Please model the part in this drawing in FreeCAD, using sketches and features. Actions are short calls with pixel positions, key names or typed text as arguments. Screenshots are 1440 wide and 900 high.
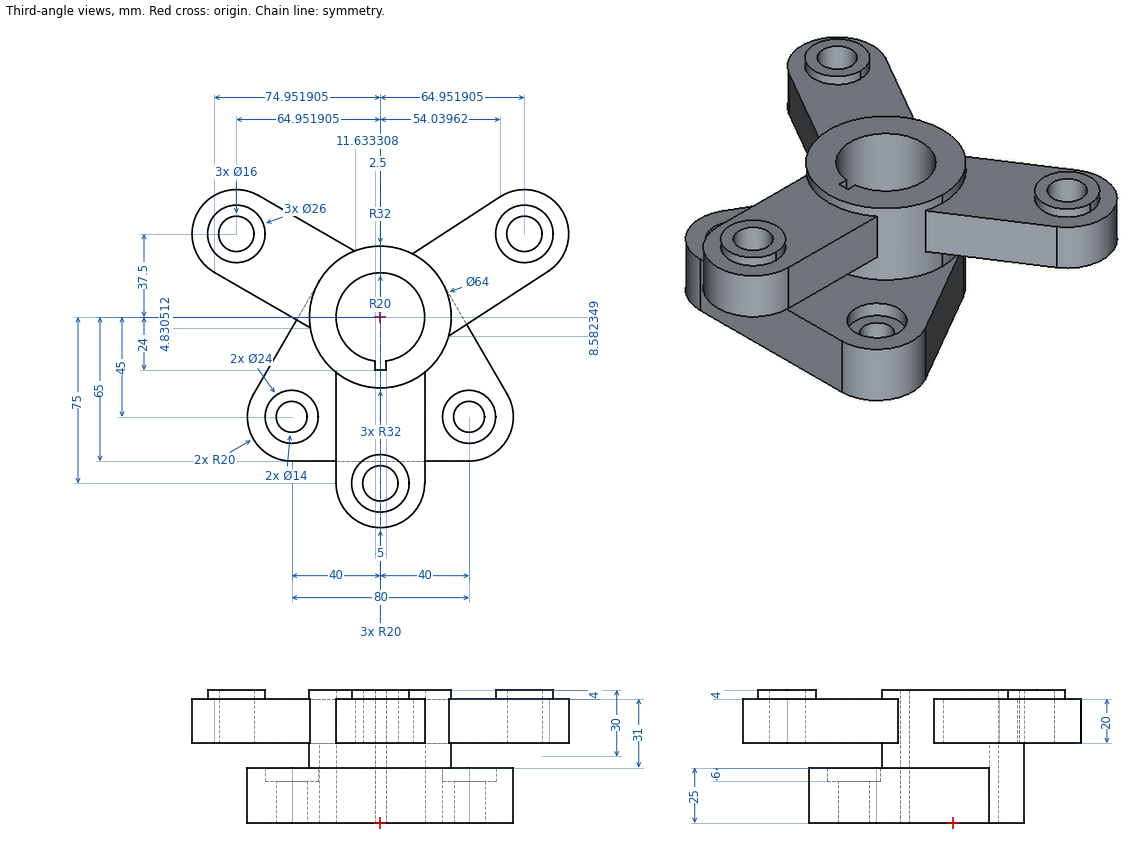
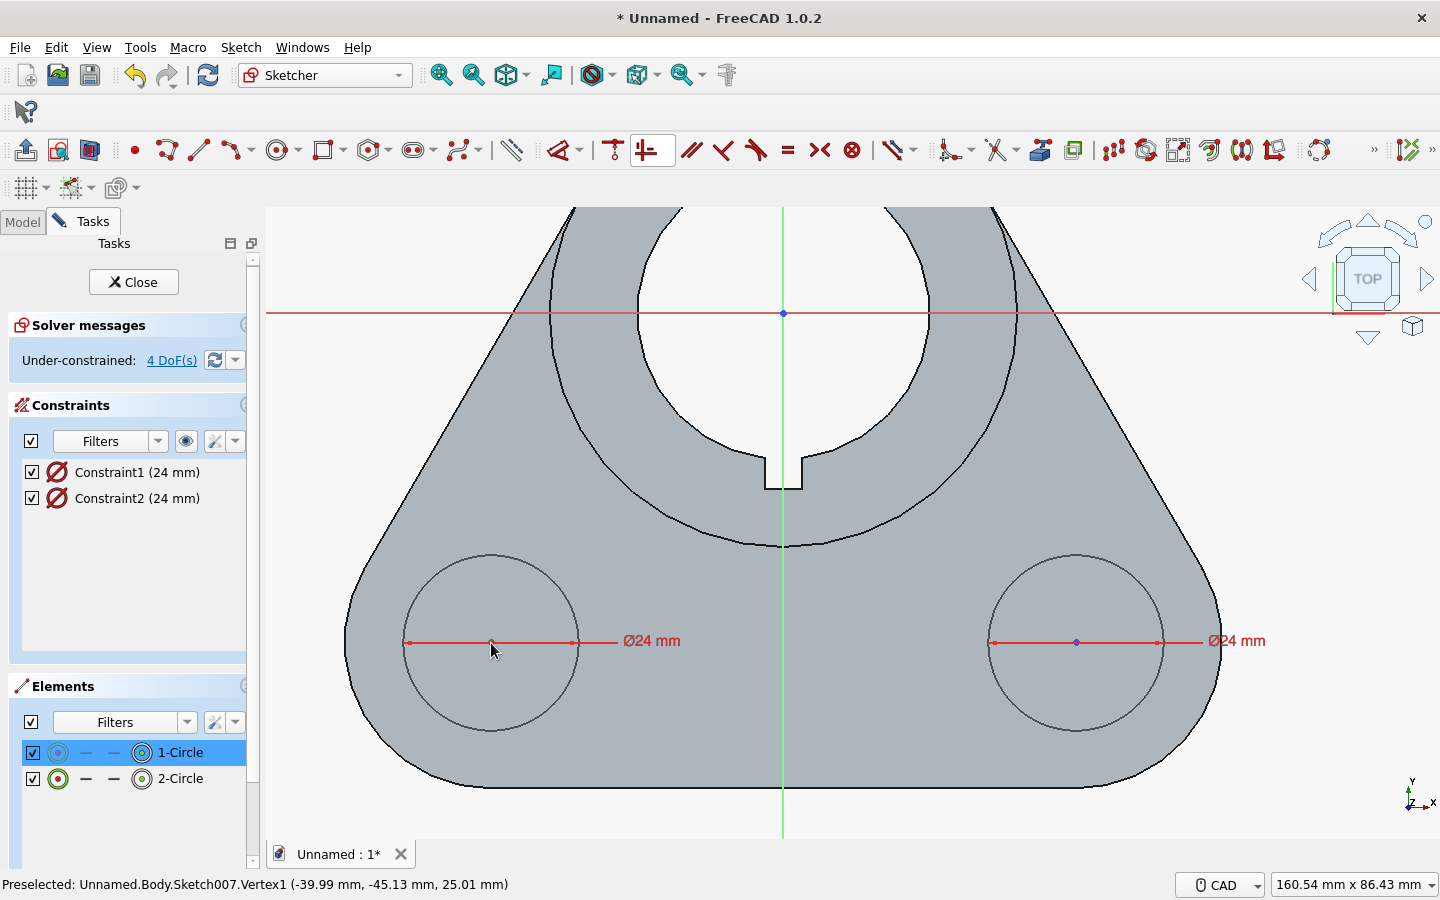
click(1076, 643)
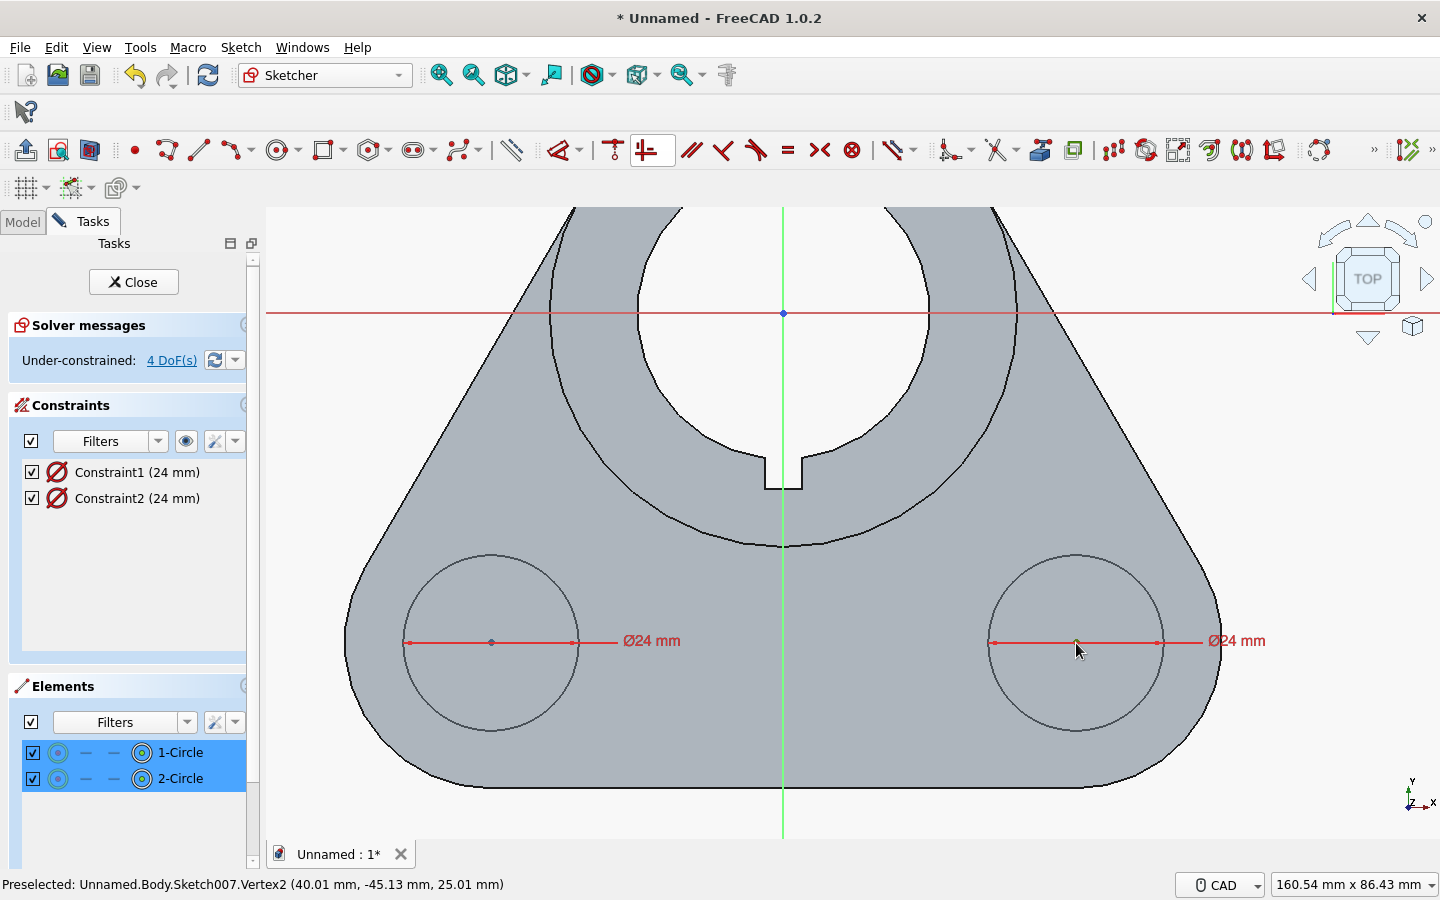
click(670, 150)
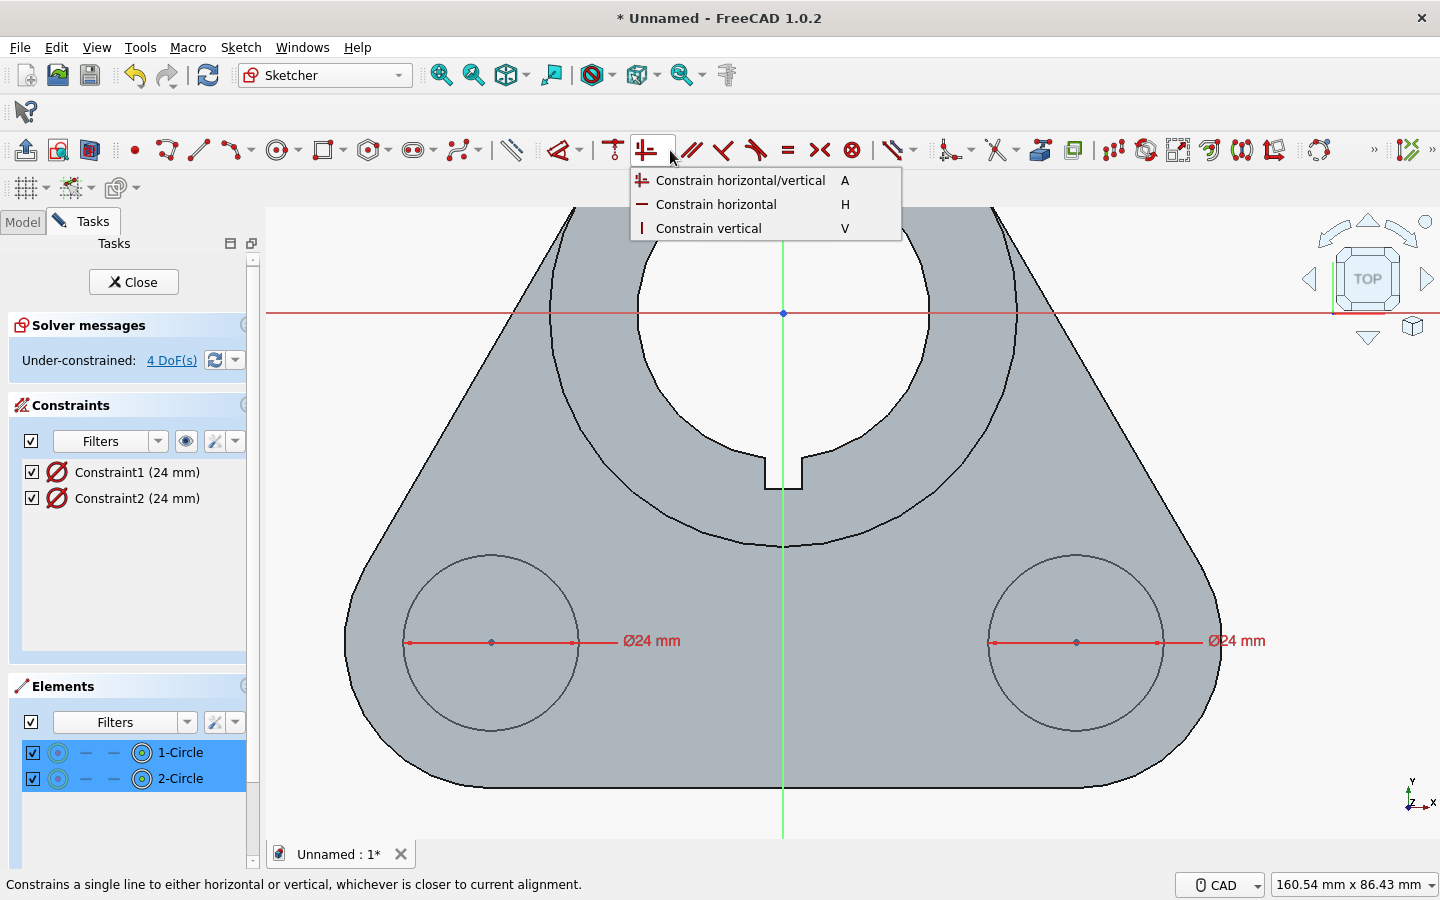
click(766, 204)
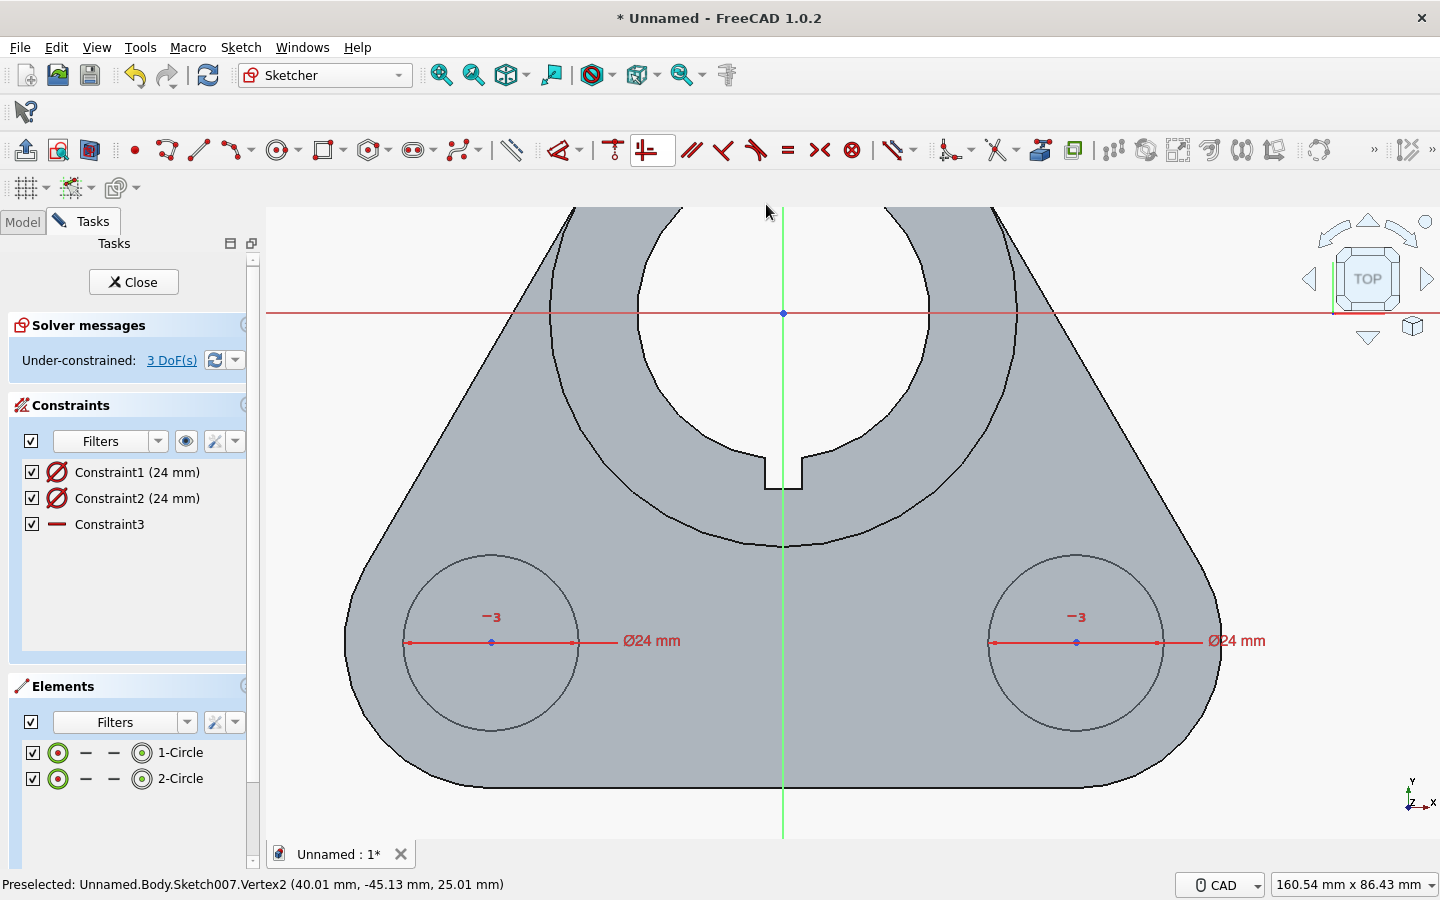
click(558, 150)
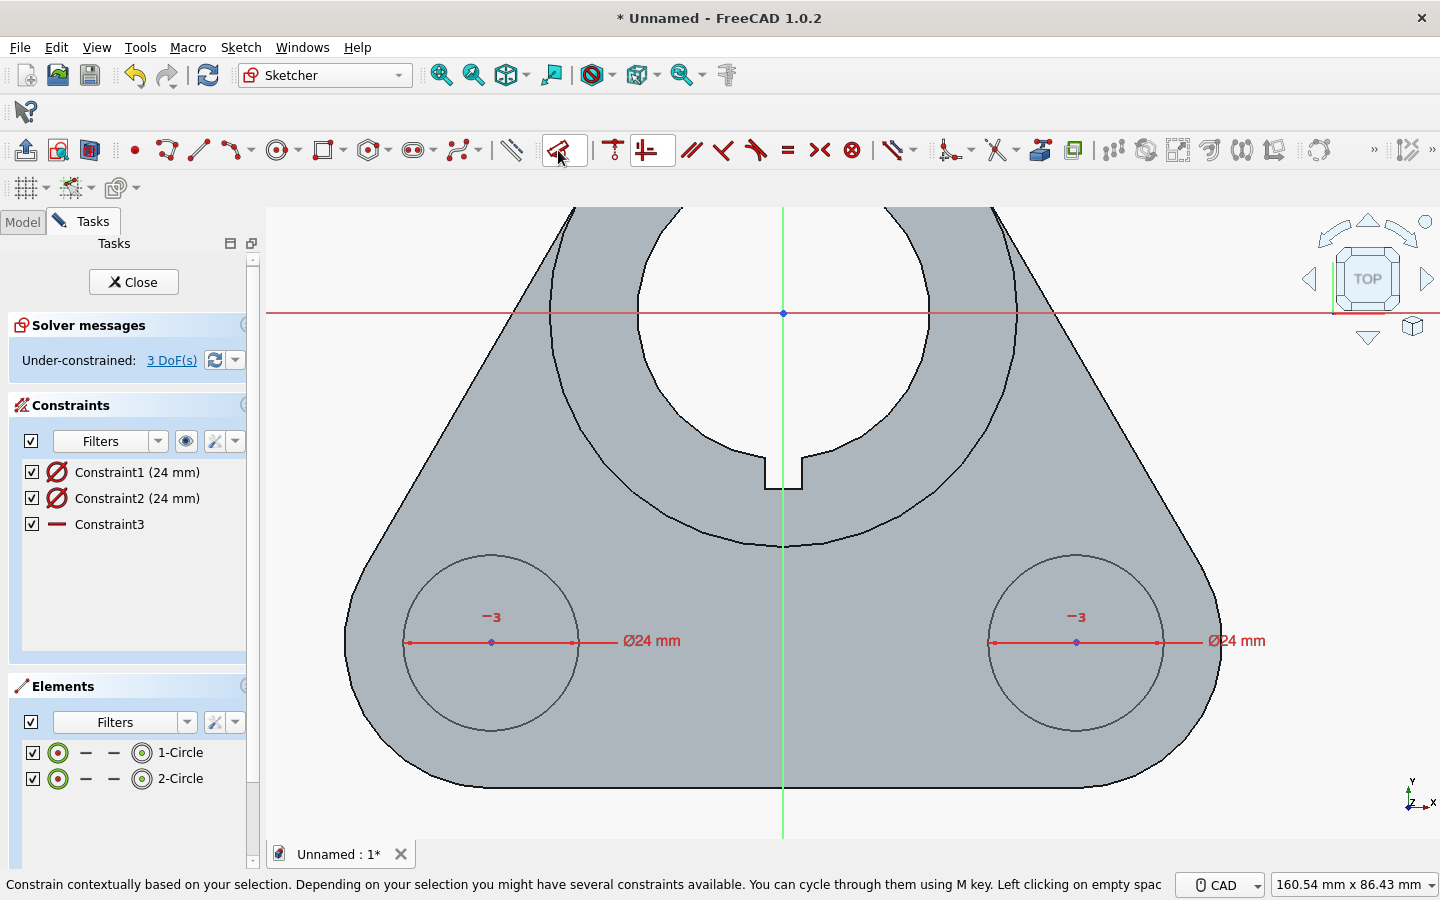
click(491, 643)
click(637, 279)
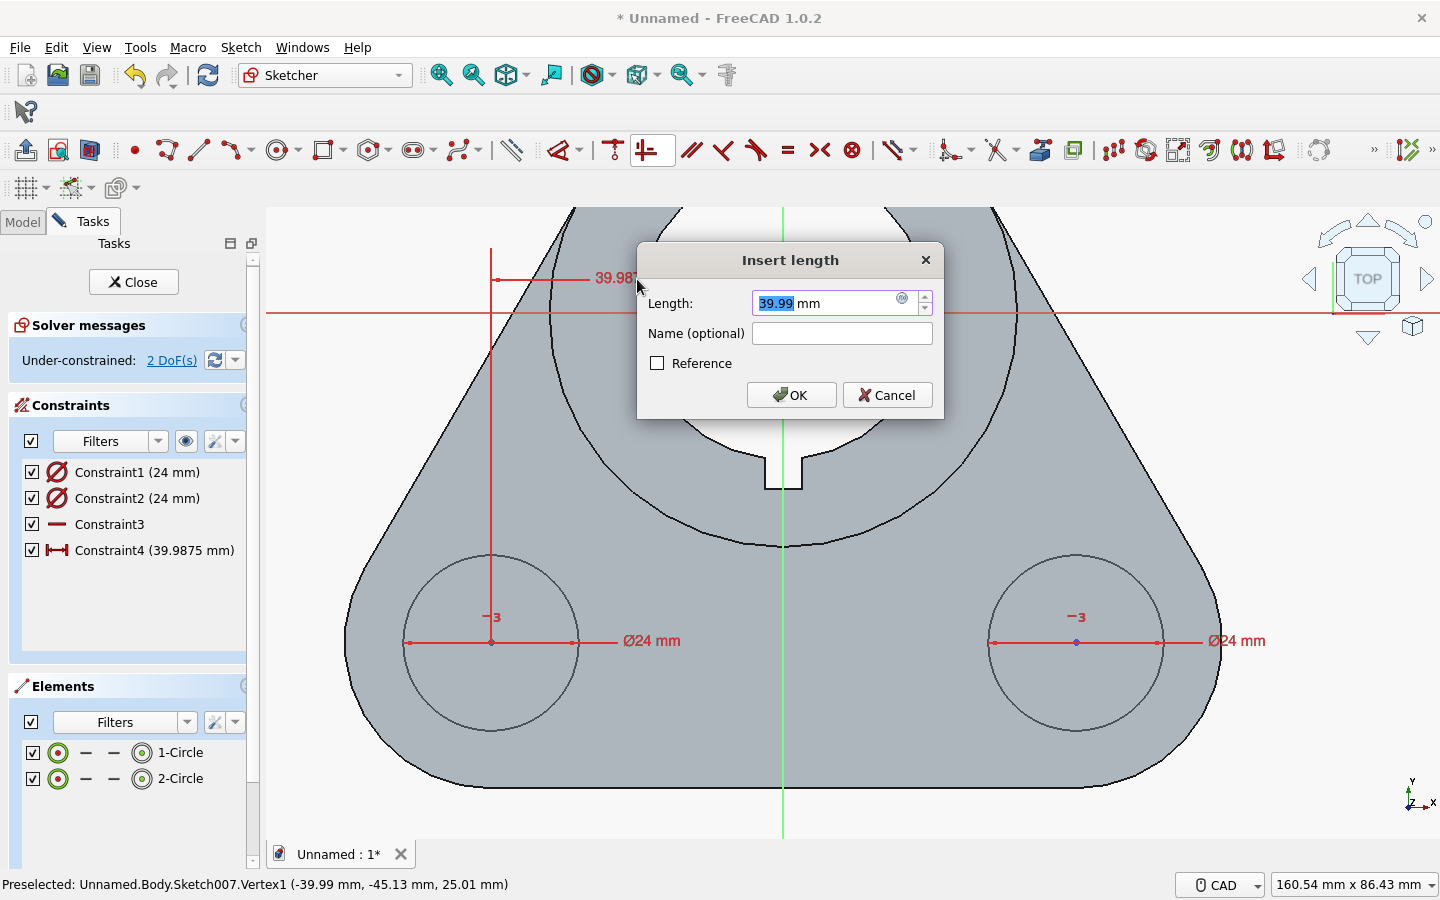
text(40)
key(Return)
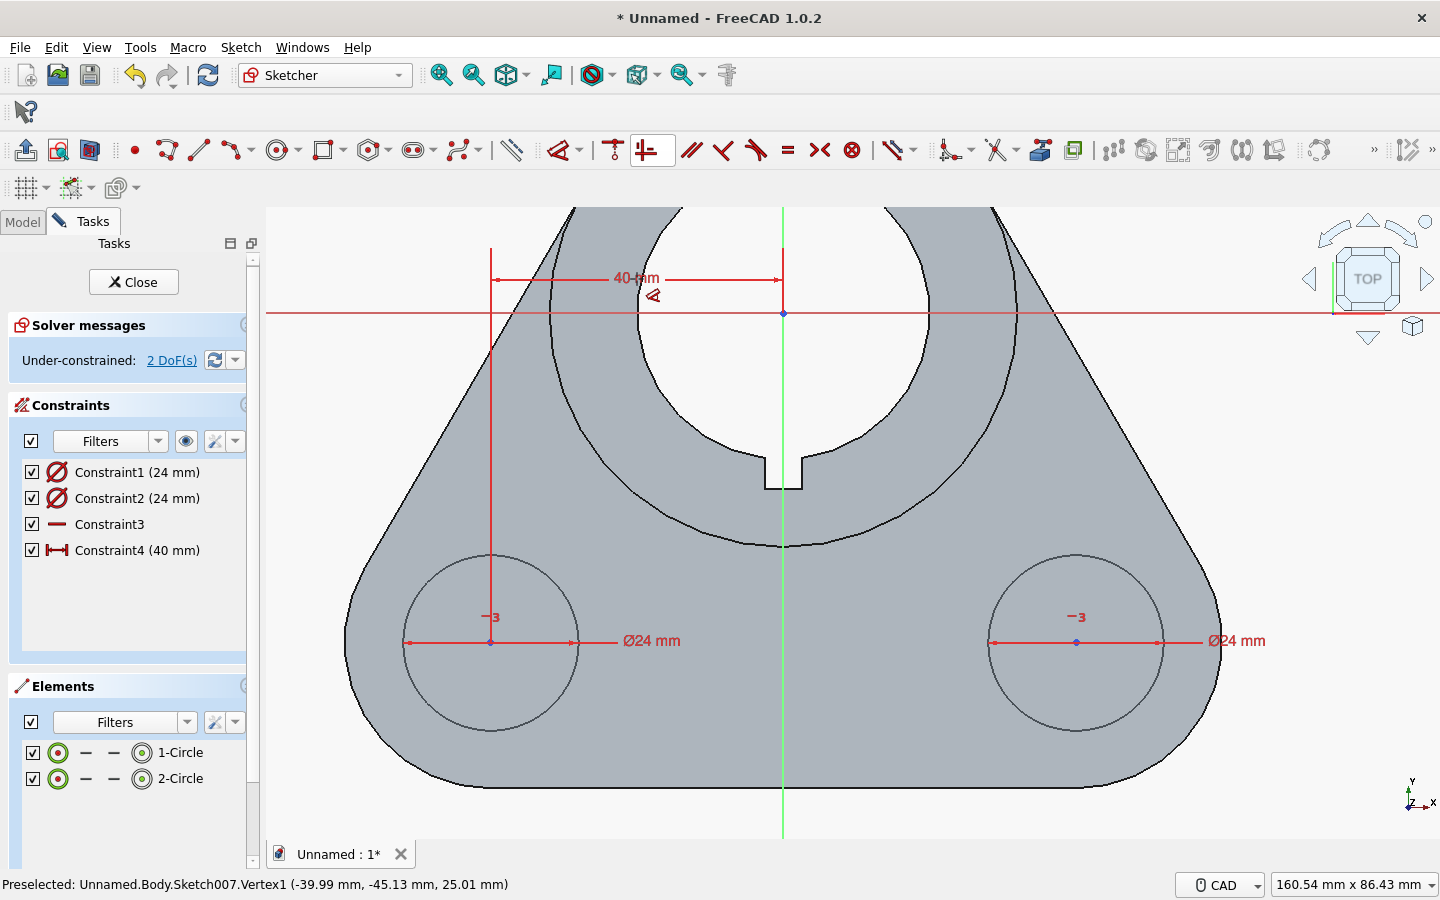
click(491, 643)
click(457, 478)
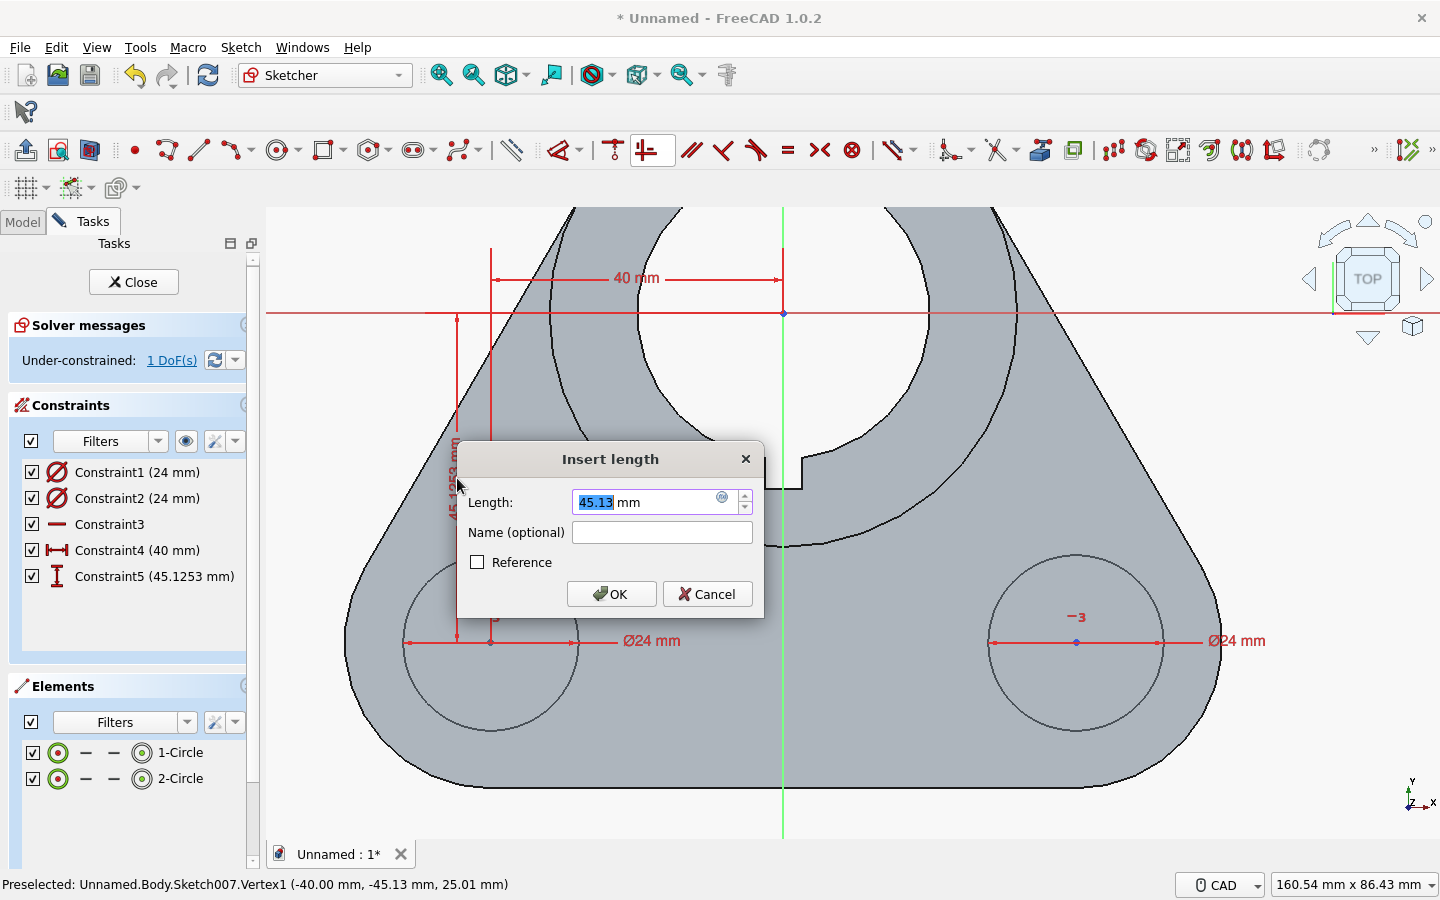
text(45)
key(Return)